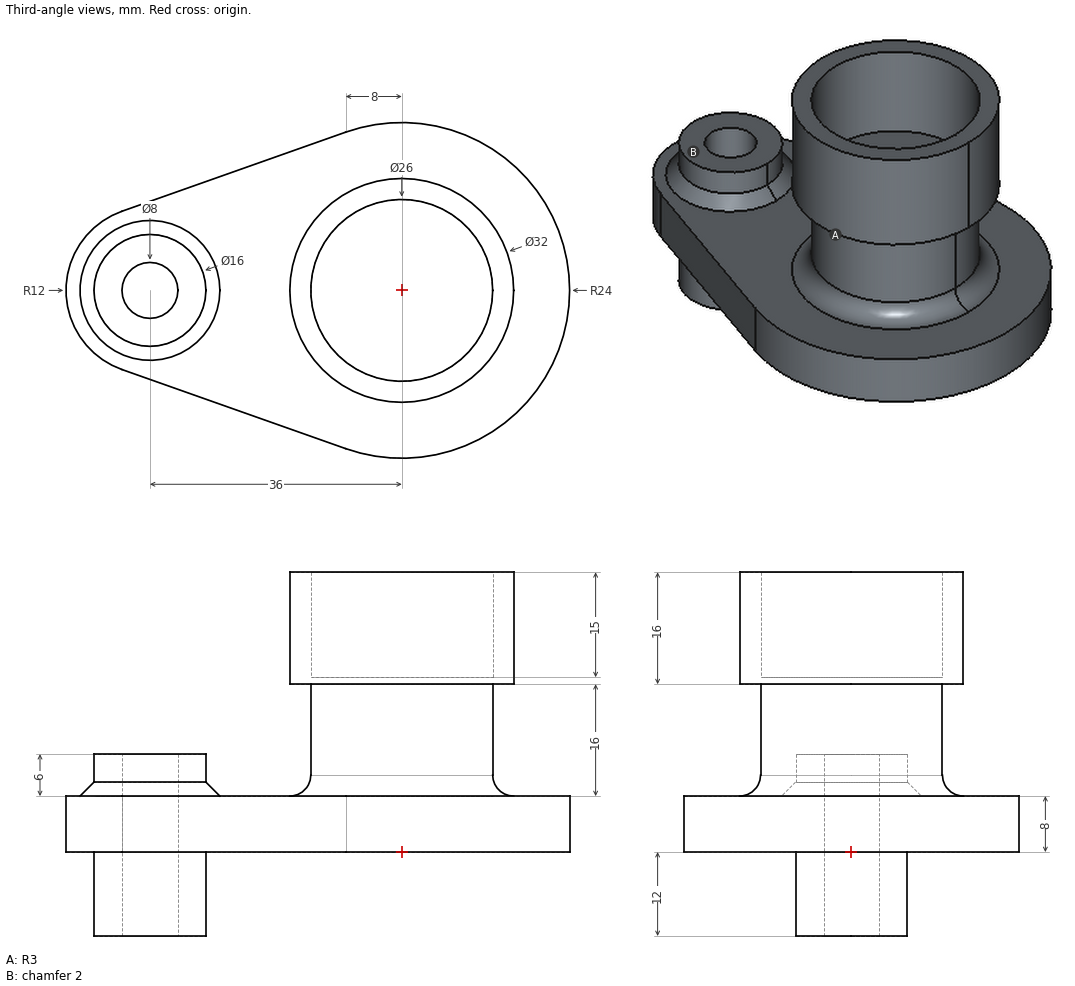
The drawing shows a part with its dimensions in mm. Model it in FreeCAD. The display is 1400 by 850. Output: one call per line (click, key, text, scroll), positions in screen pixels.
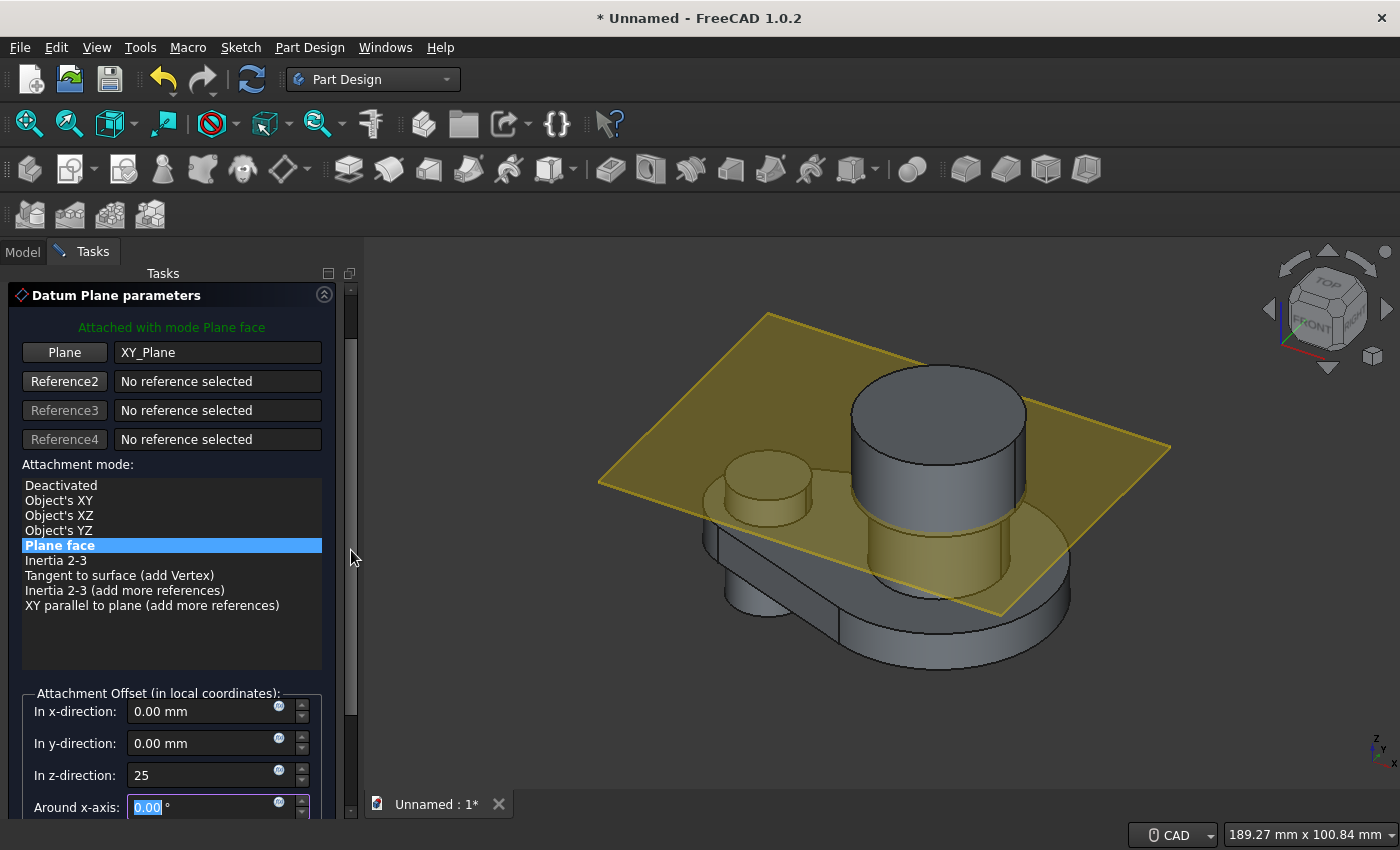
click(124, 312)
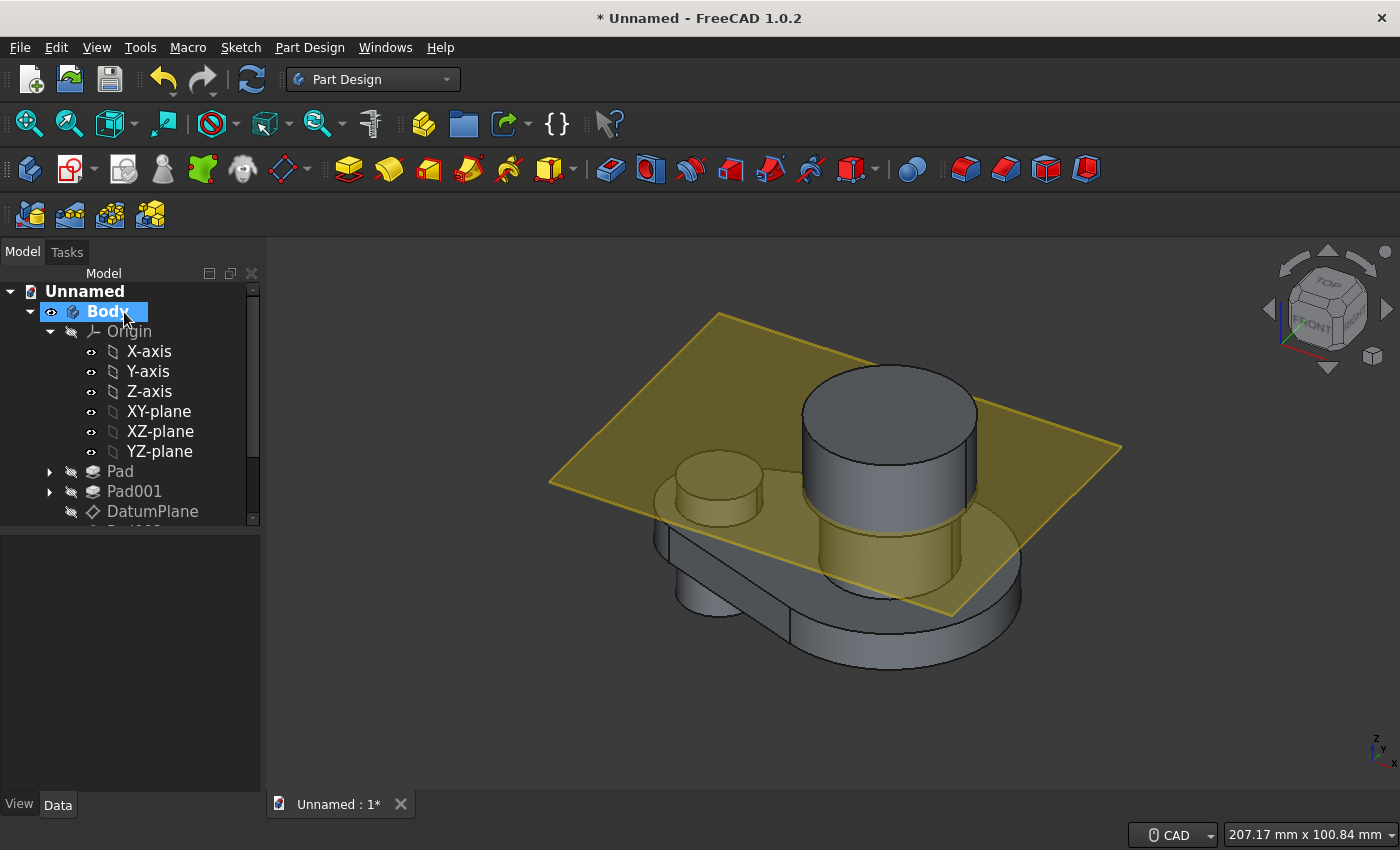
scroll(100, 407, down, 3)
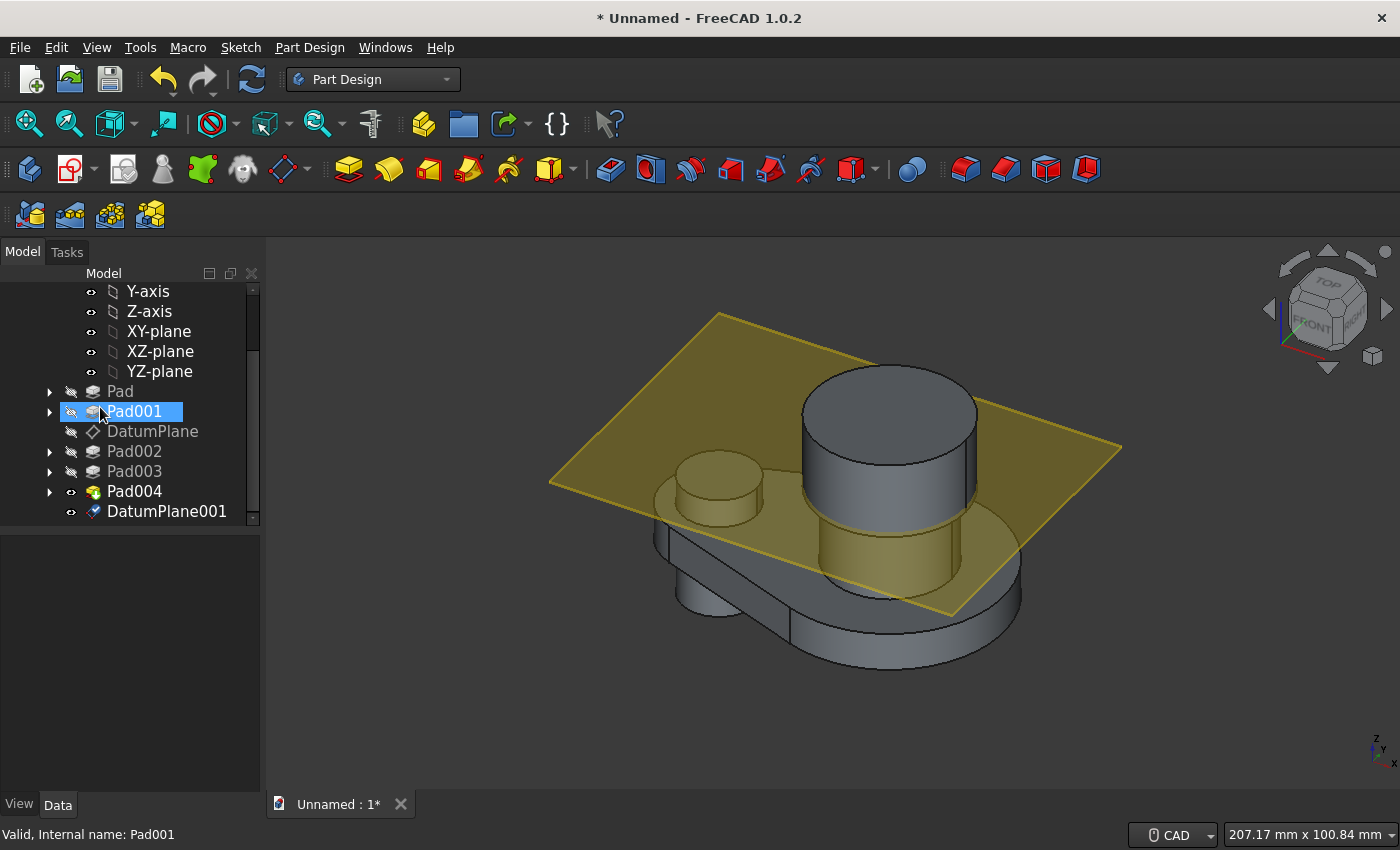
click(116, 512)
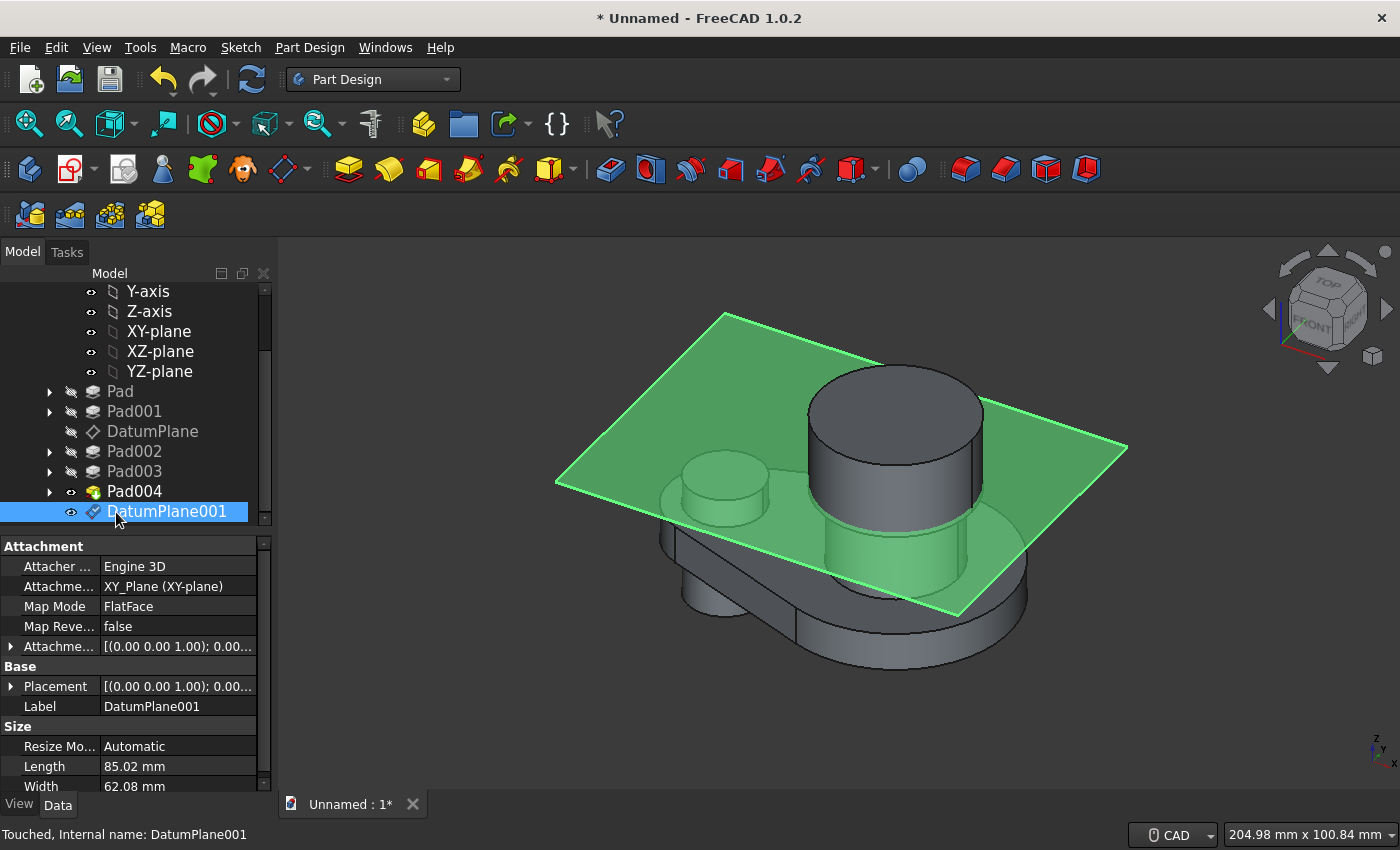
click(70, 170)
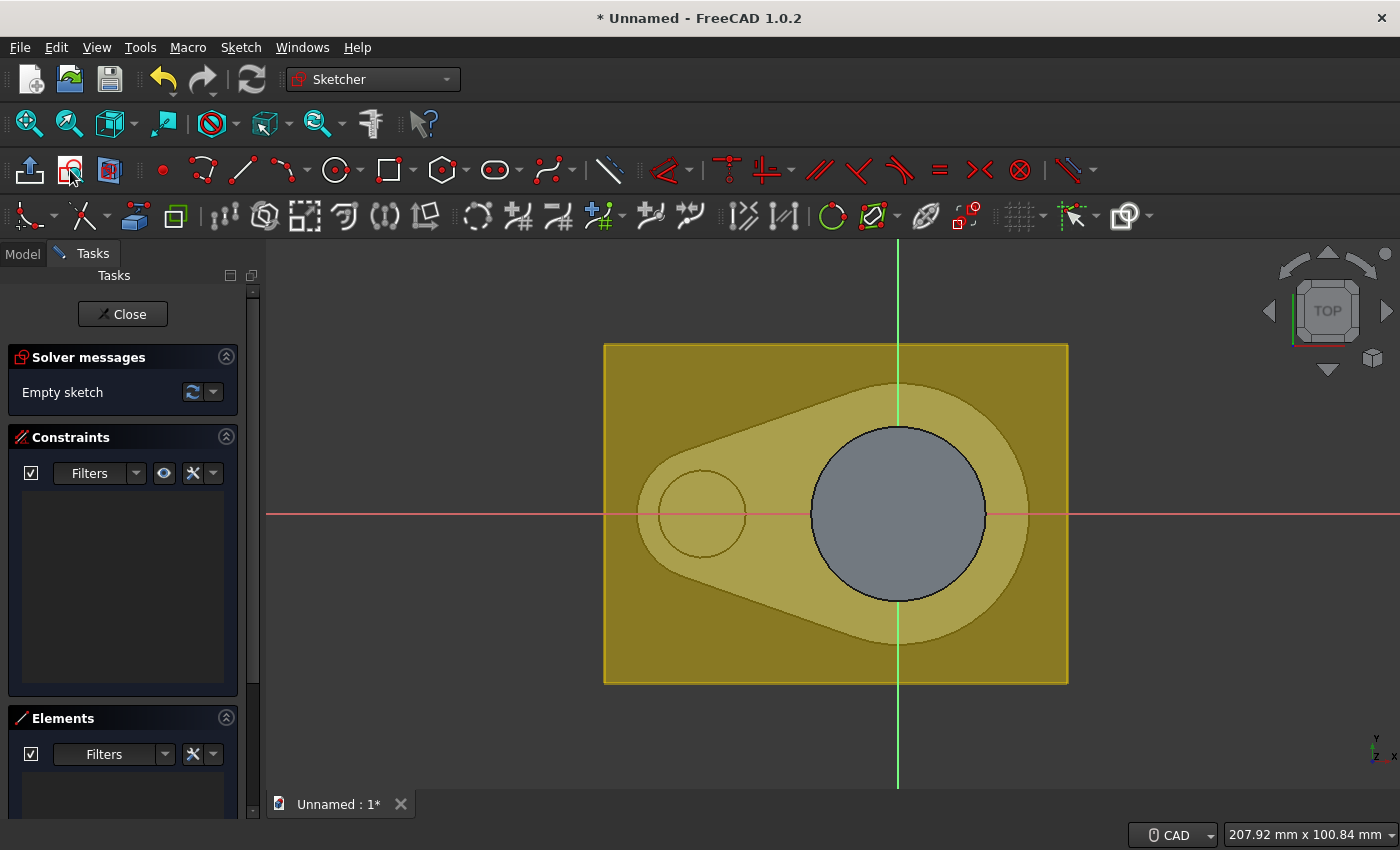
click(110, 170)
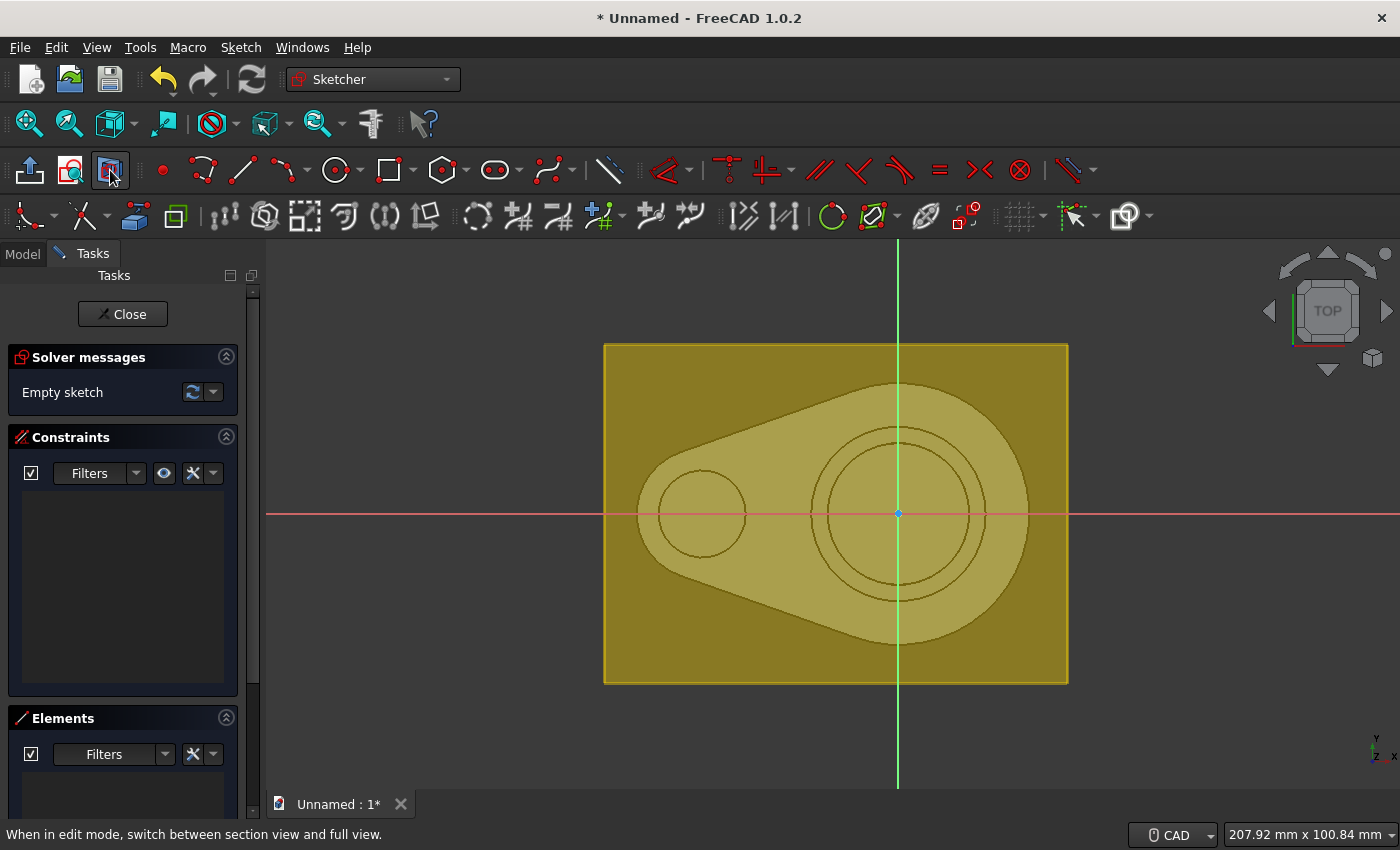
scroll(1008, 514, up, 4)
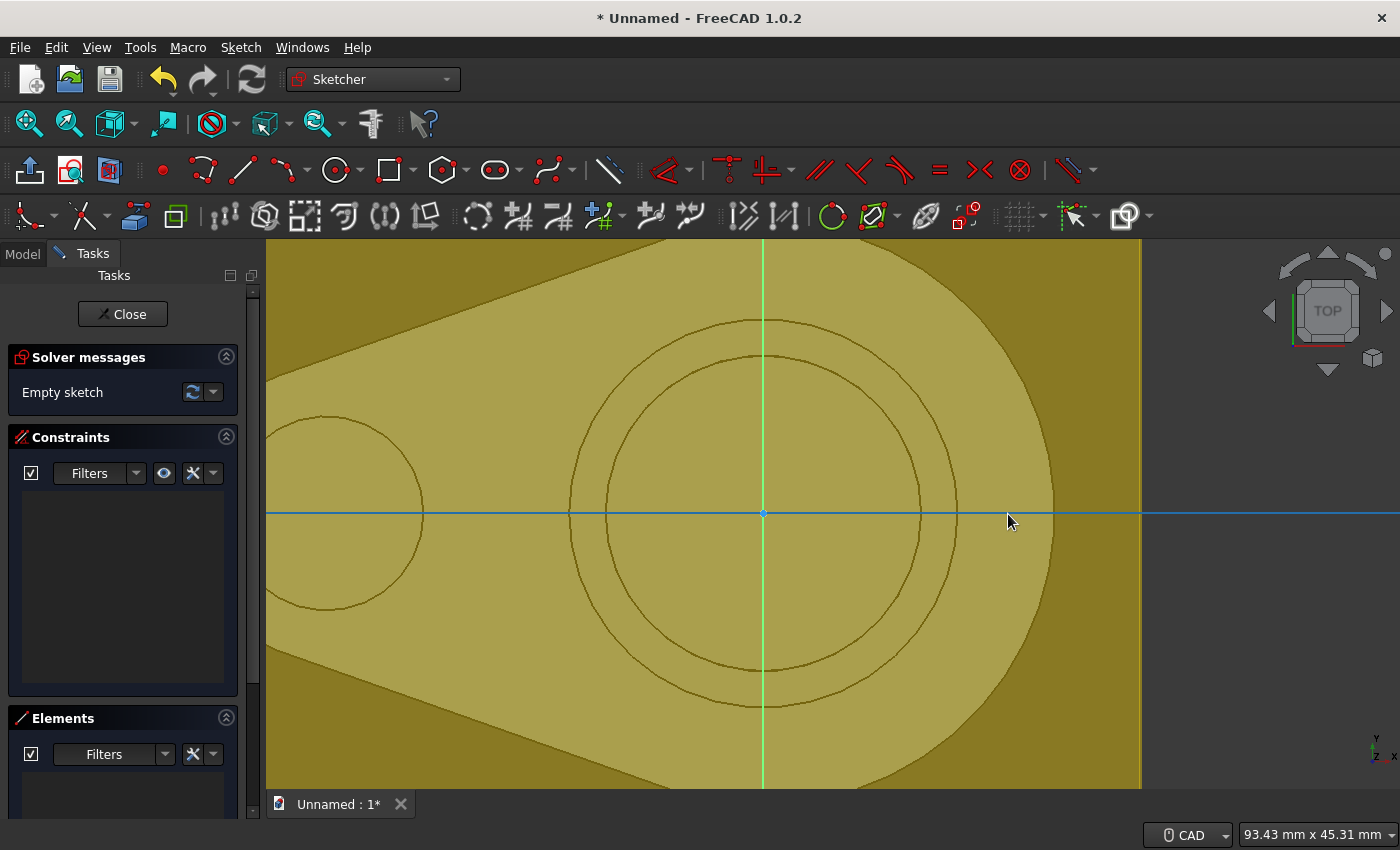
click(336, 170)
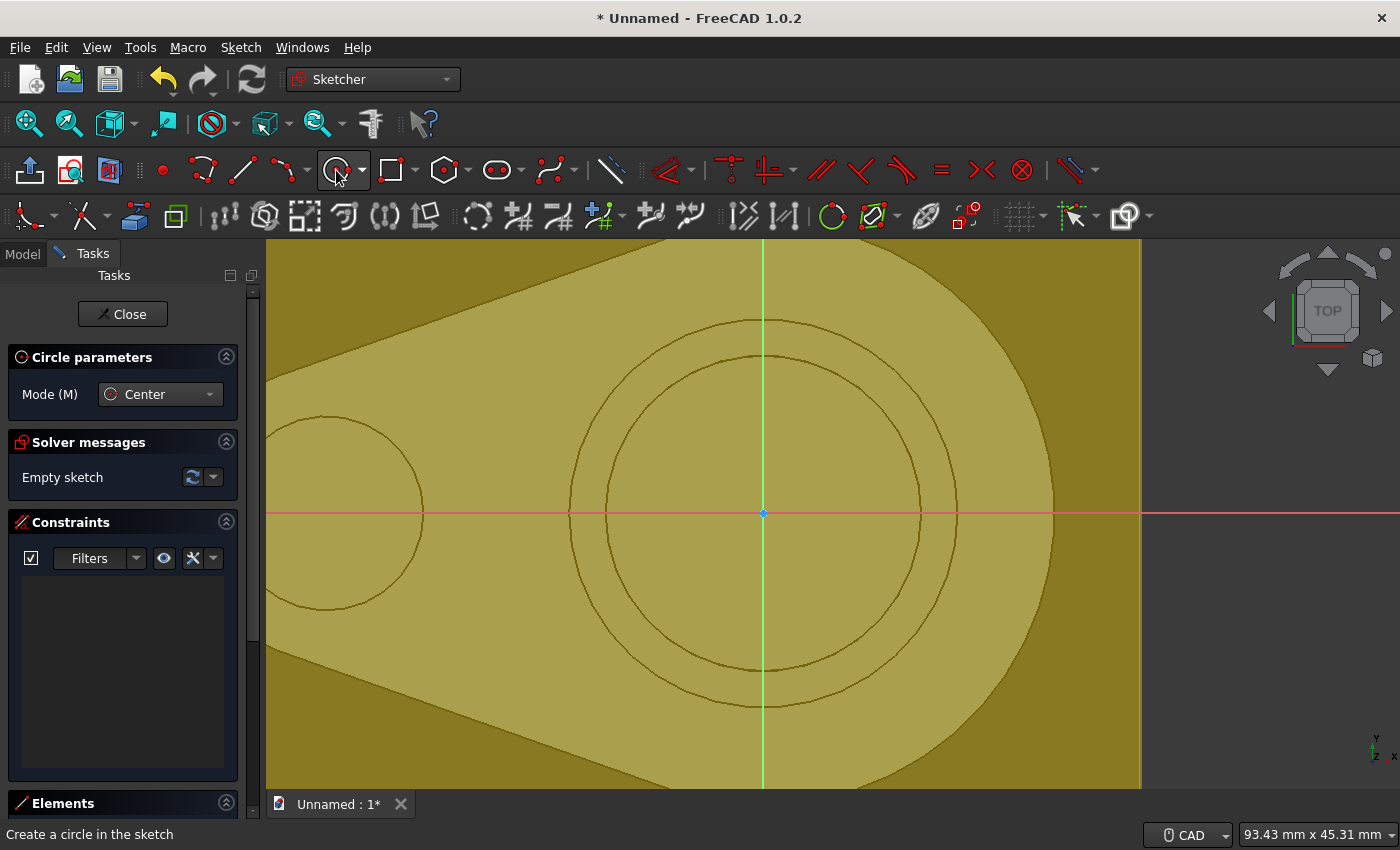
click(763, 513)
move(875, 402)